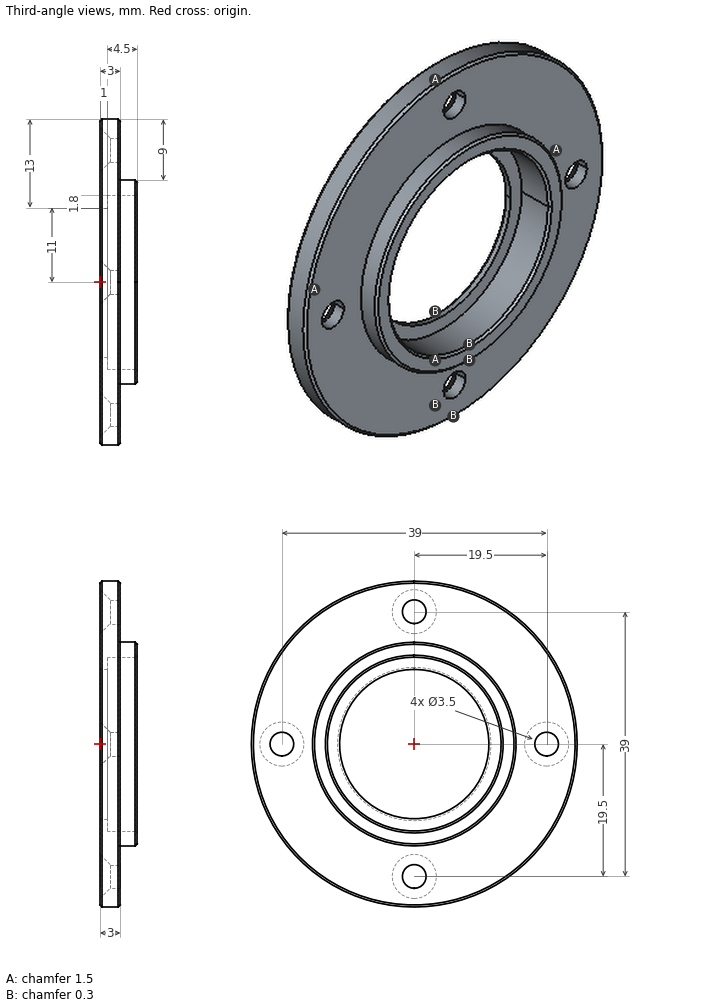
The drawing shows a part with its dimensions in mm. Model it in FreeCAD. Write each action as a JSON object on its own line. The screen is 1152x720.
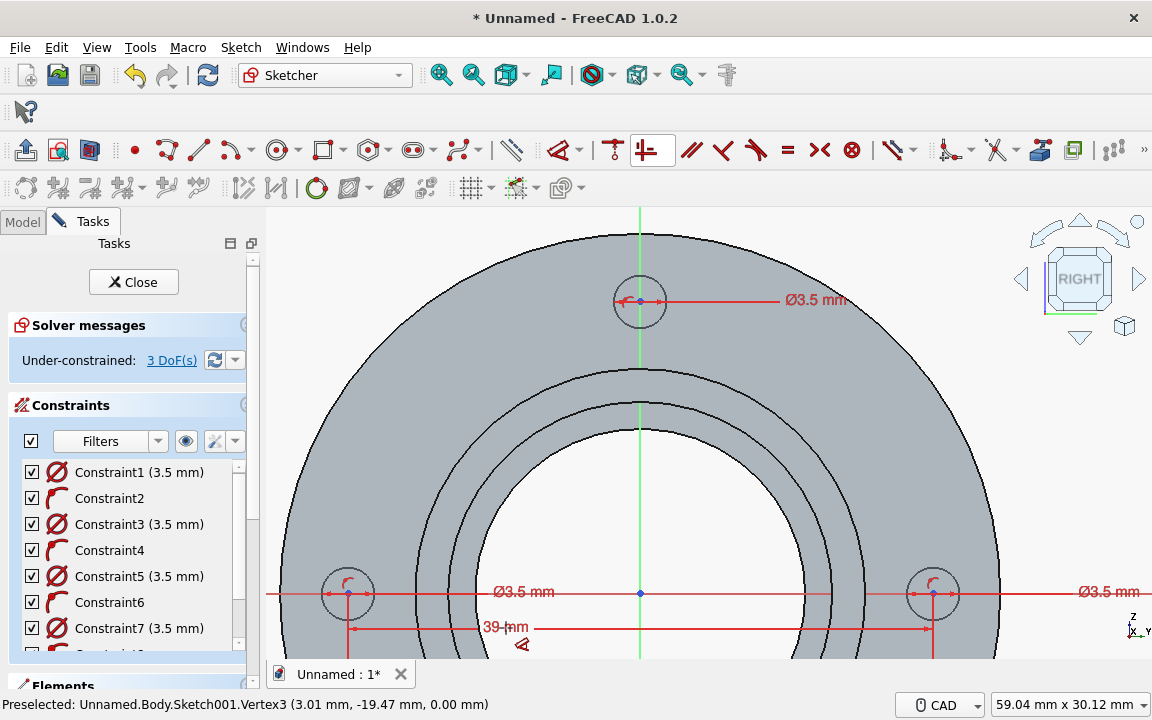
{"action": "scroll", "coordinate": [641, 302], "scroll_direction": "down", "scroll_amount": 4}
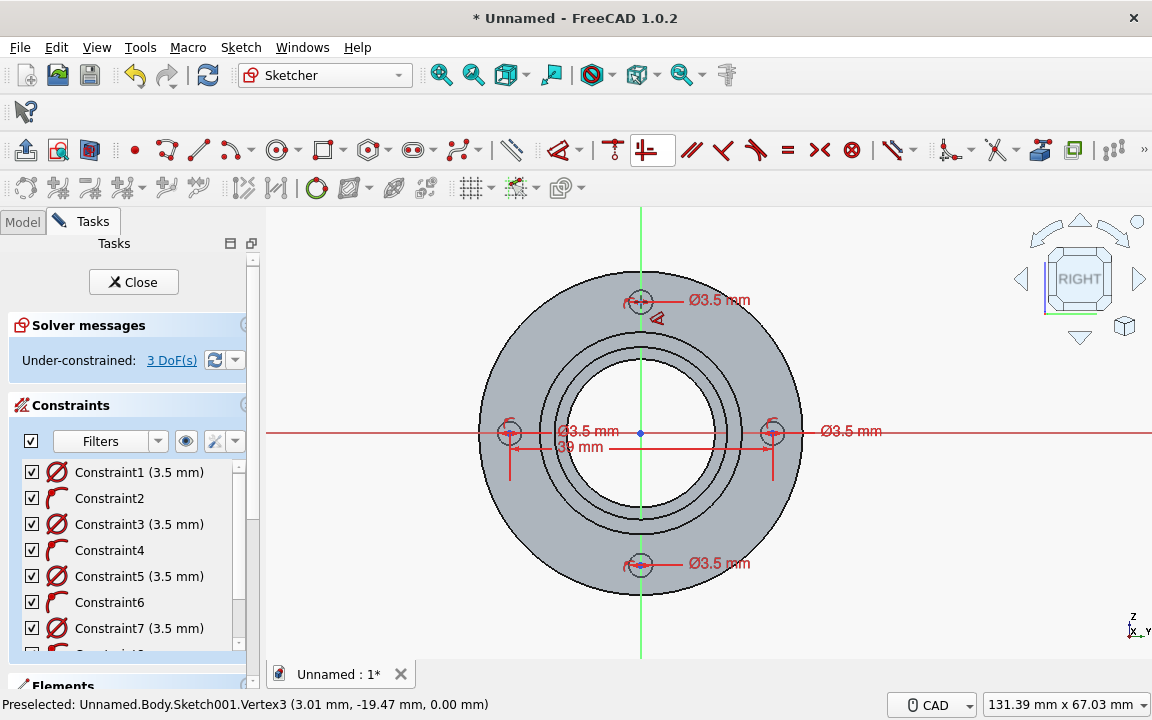
{"action": "left_click", "coordinate": [641, 565]}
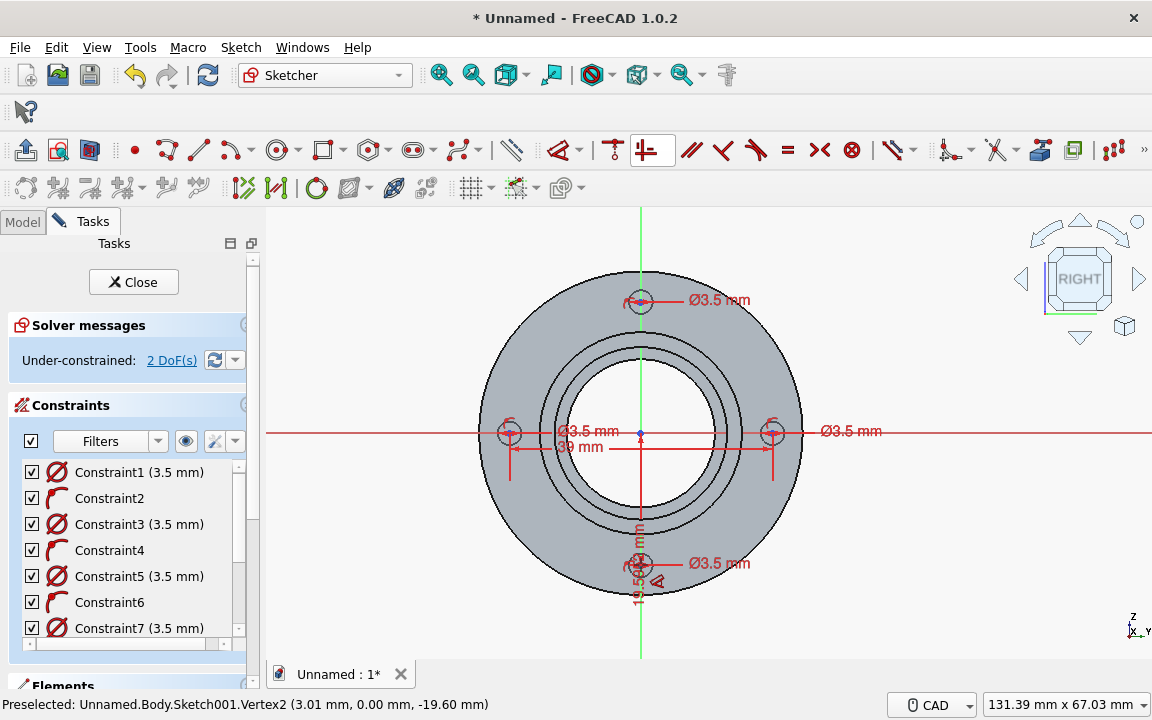
{"action": "left_click", "coordinate": [641, 302]}
{"action": "left_click", "coordinate": [675, 373]}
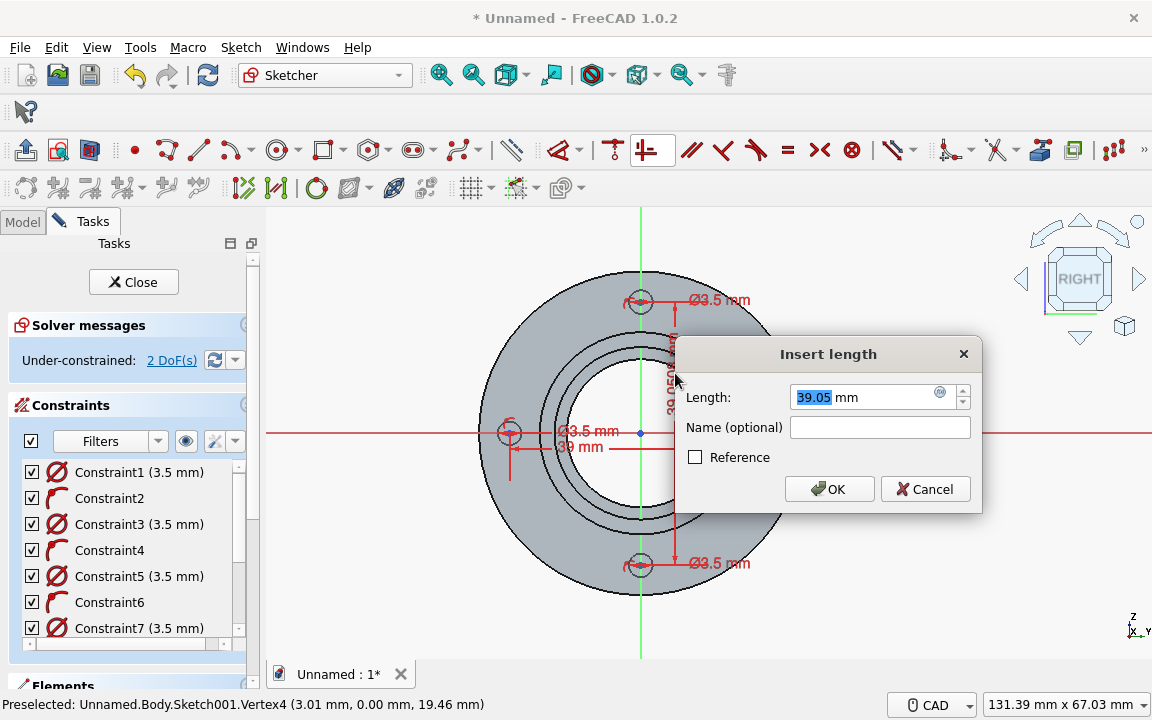
{"action": "type", "text": "39"}
{"action": "key", "text": "Return"}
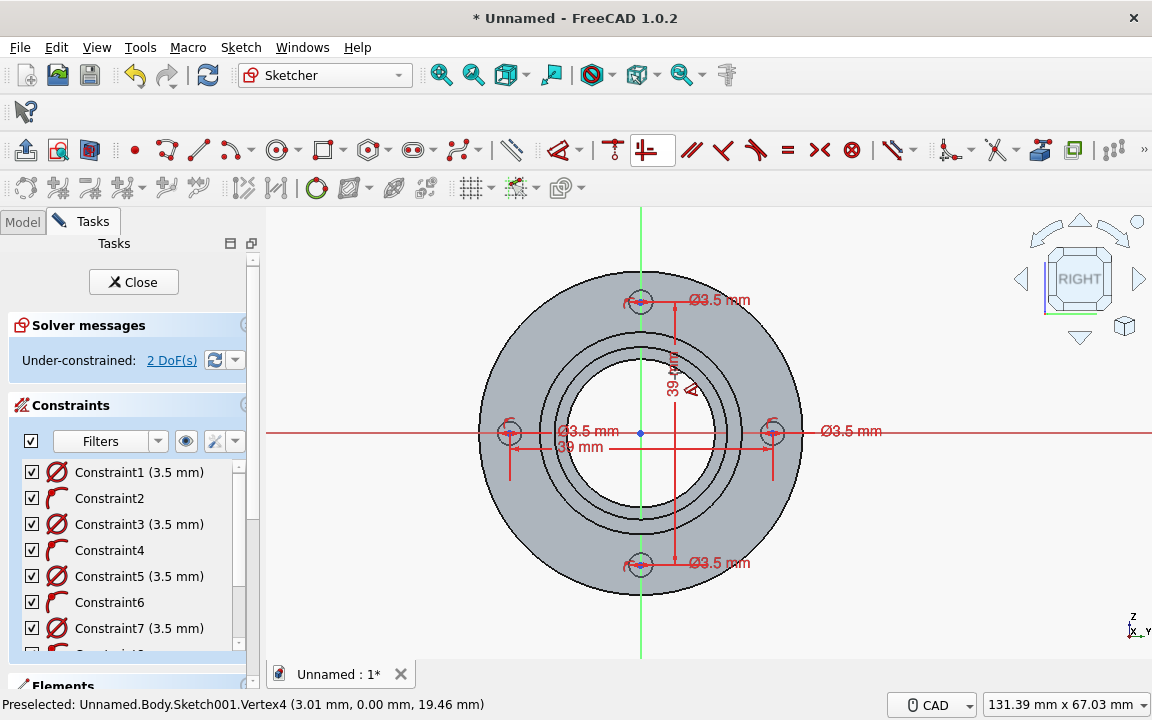
{"action": "left_click", "coordinate": [773, 433]}
{"action": "left_click", "coordinate": [707, 467]}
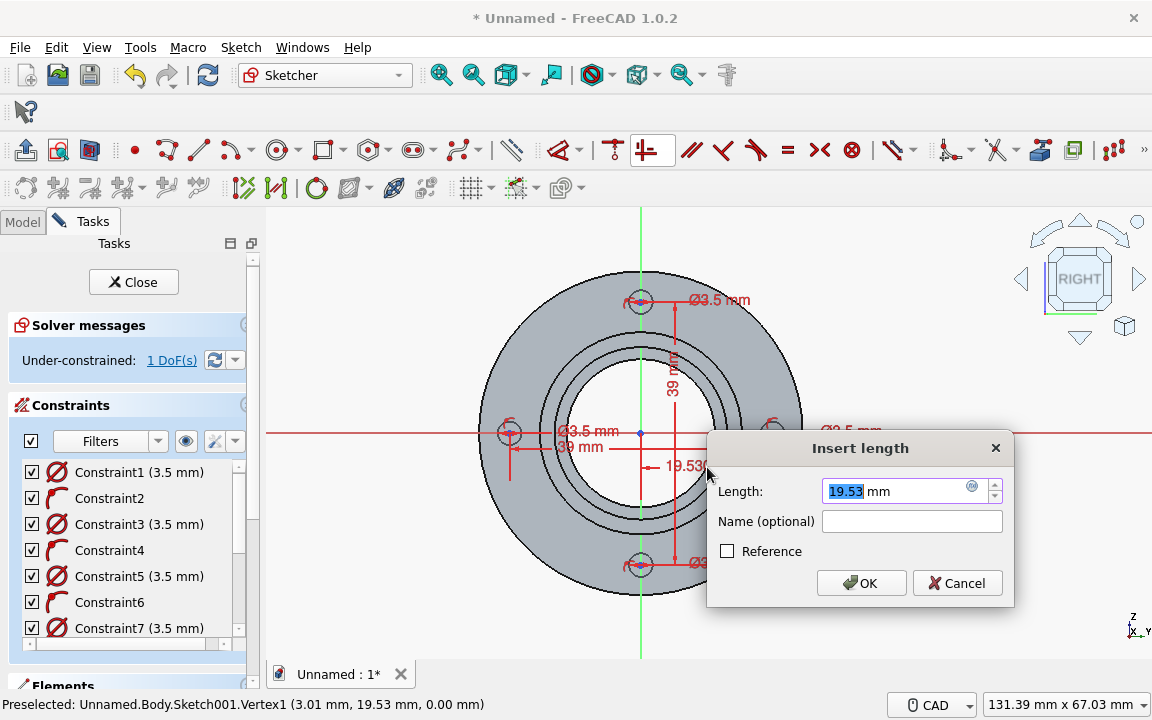
{"action": "type", "text": "19.5"}
{"action": "key", "text": "Return"}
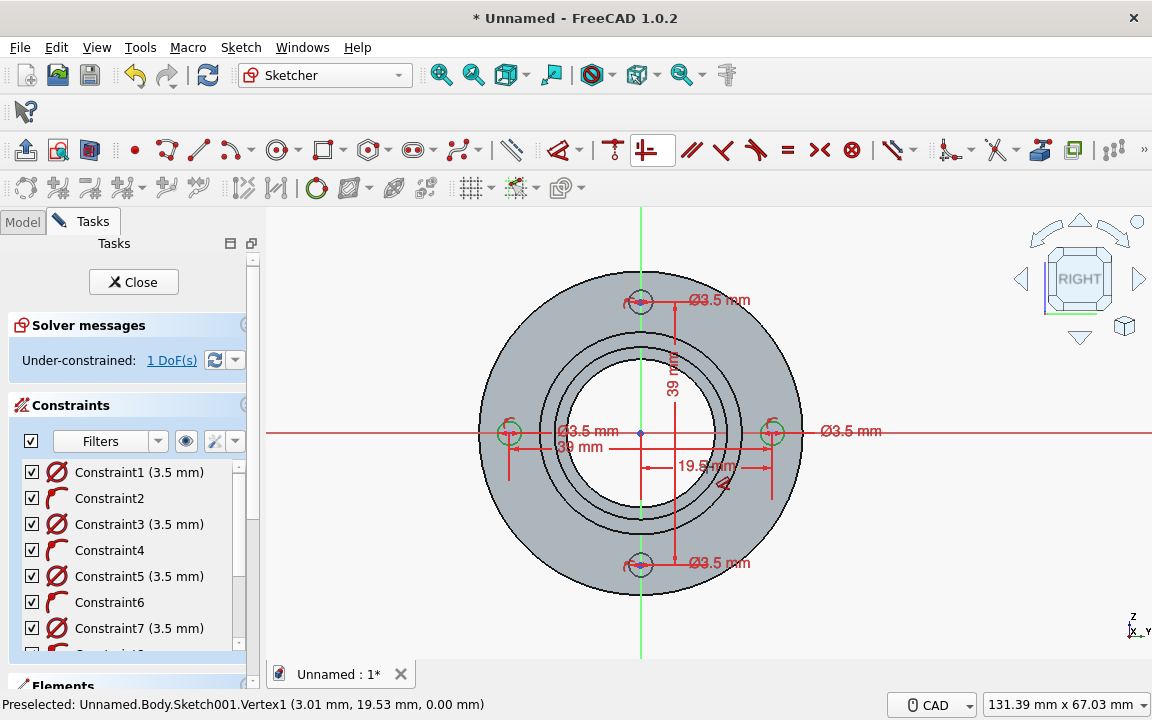
{"action": "left_click", "coordinate": [641, 565]}
{"action": "left_click", "coordinate": [675, 499]}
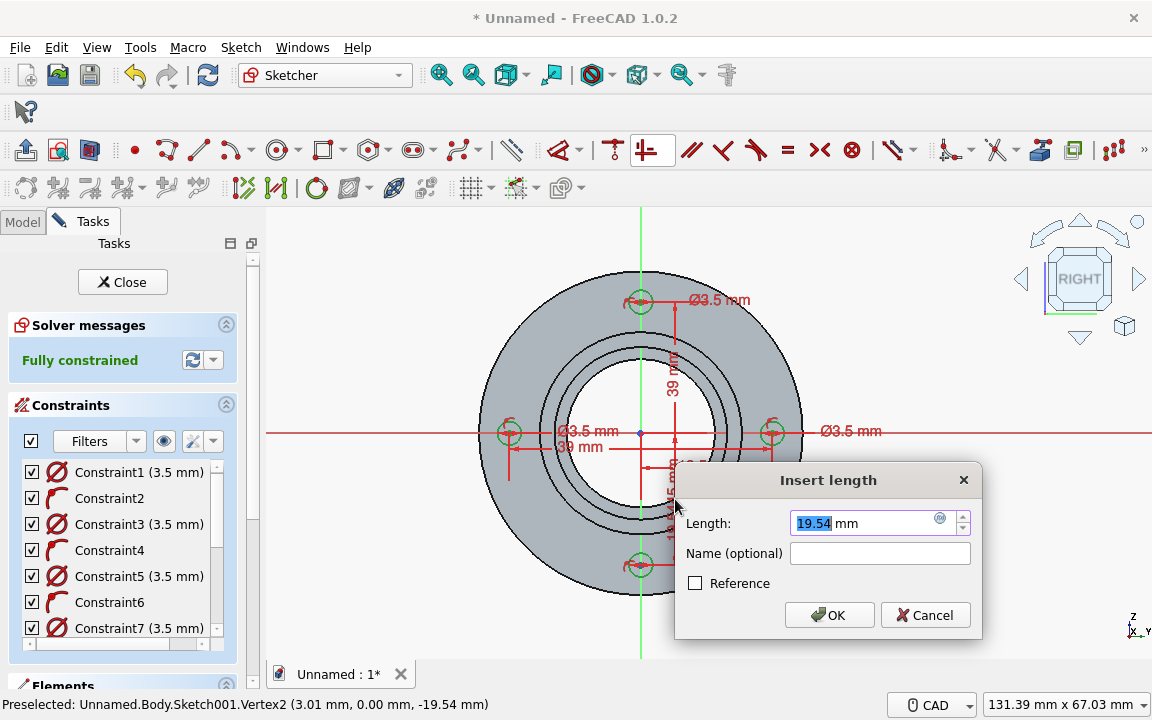
{"action": "type", "text": "19.5"}
{"action": "key", "text": "Return"}
{"action": "key", "text": "Escape"}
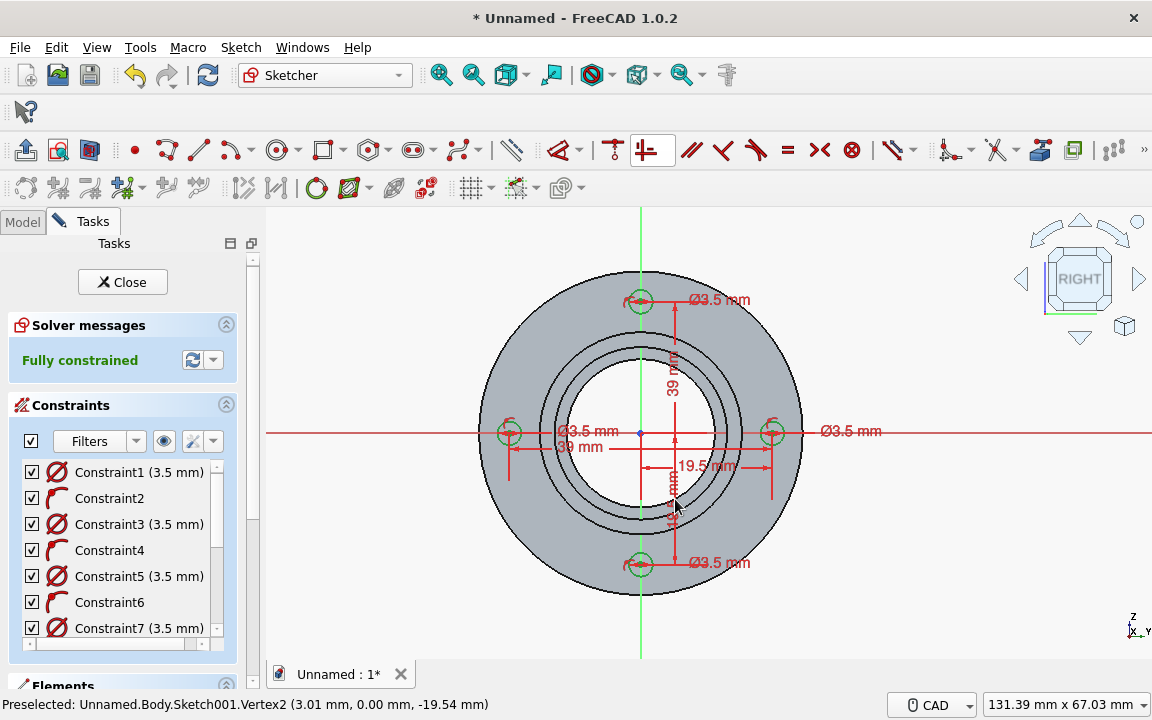
{"action": "left_click", "coordinate": [123, 282]}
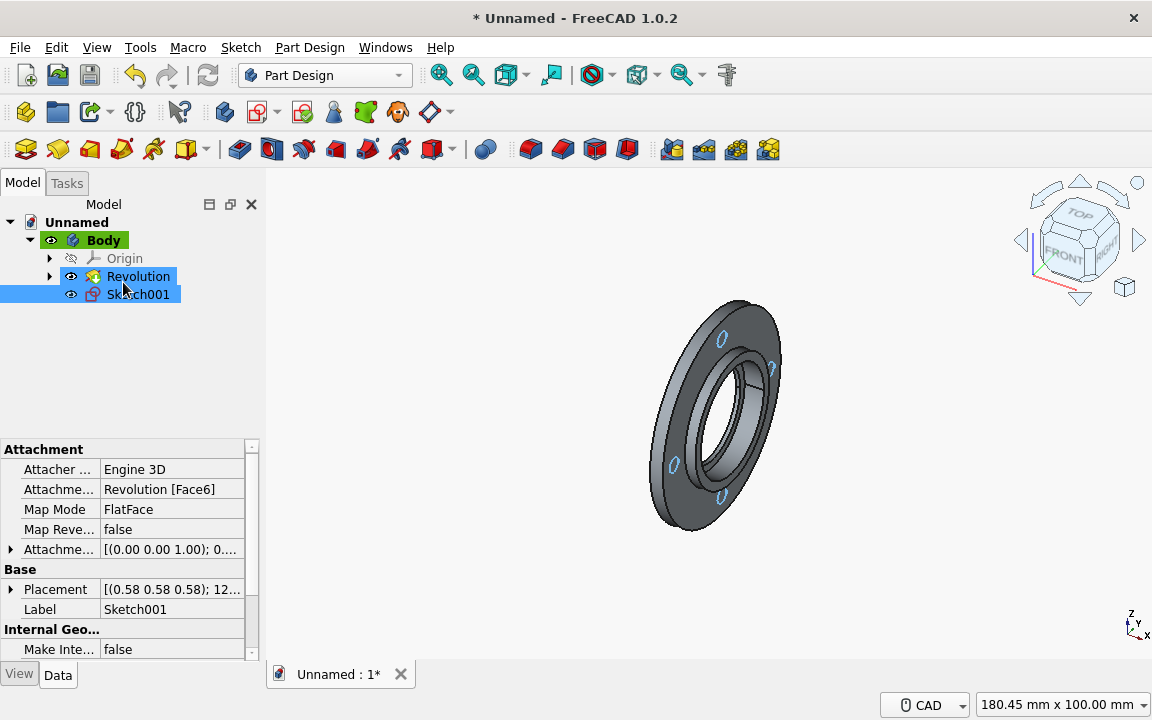
{"action": "left_click", "coordinate": [240, 150]}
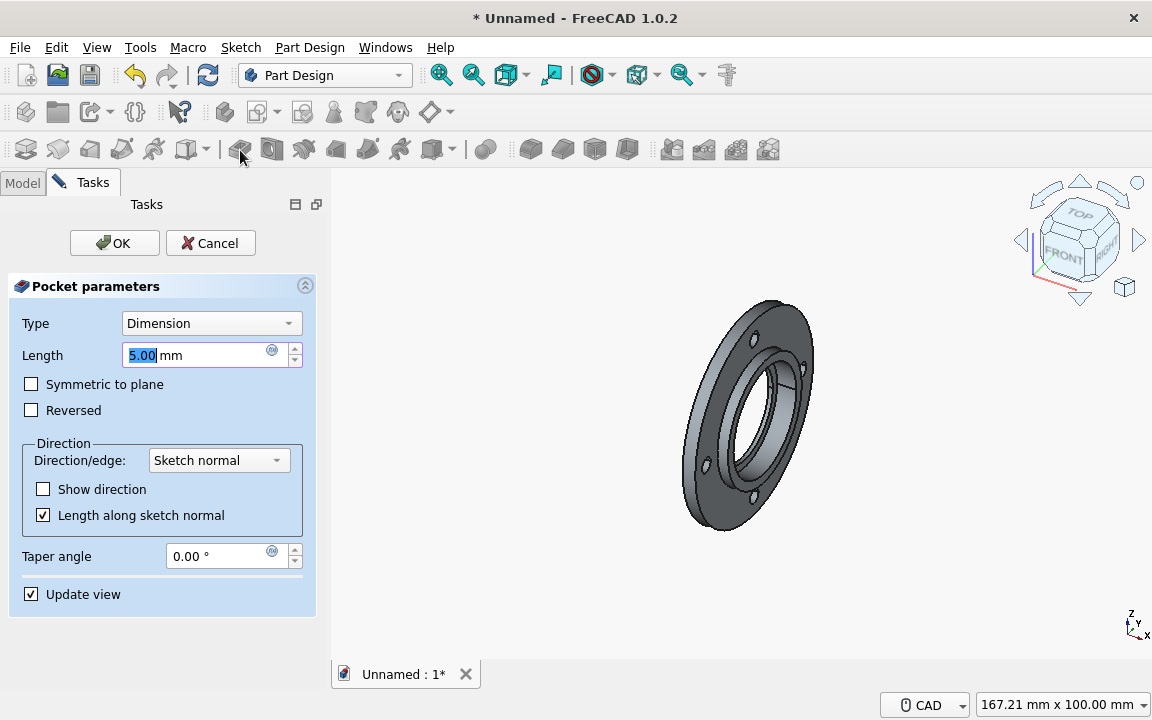
{"action": "type", "text": "3"}
{"action": "key", "text": "Tab"}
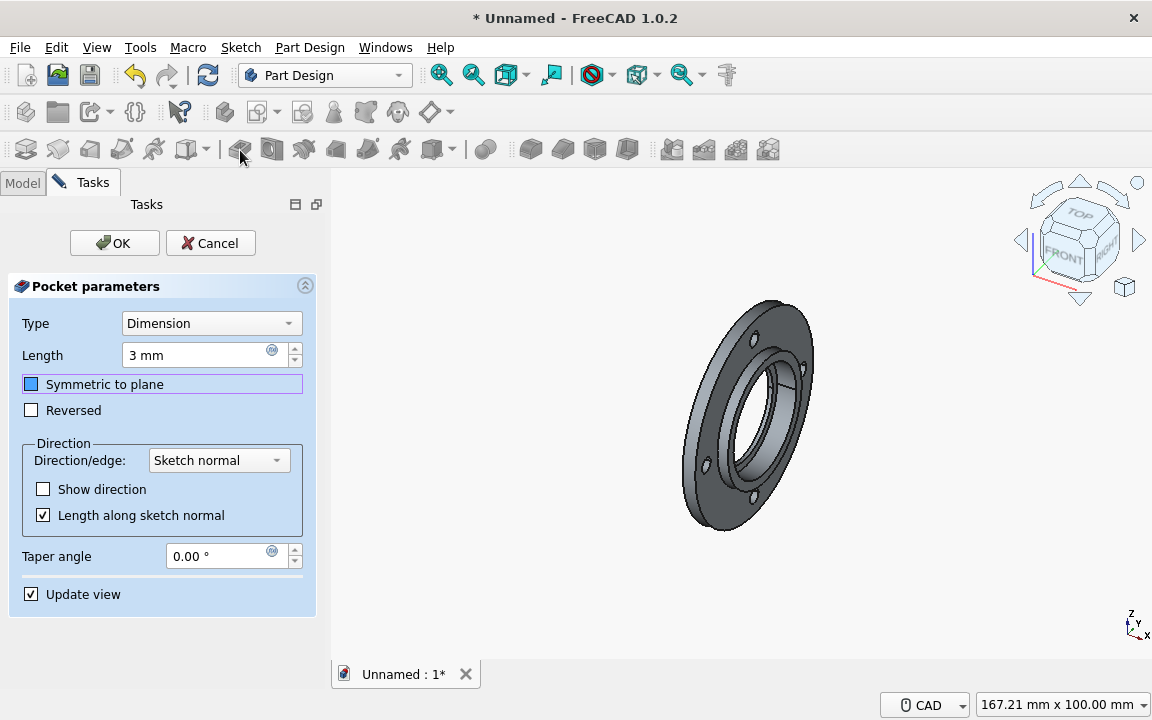
{"action": "left_click", "coordinate": [115, 243]}